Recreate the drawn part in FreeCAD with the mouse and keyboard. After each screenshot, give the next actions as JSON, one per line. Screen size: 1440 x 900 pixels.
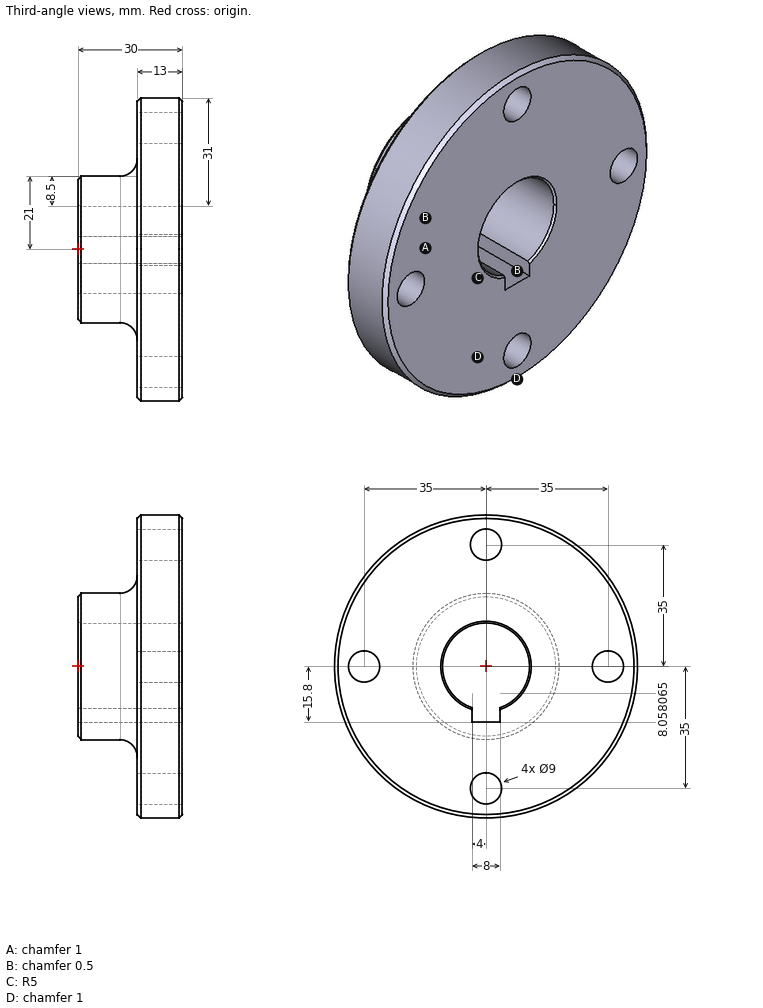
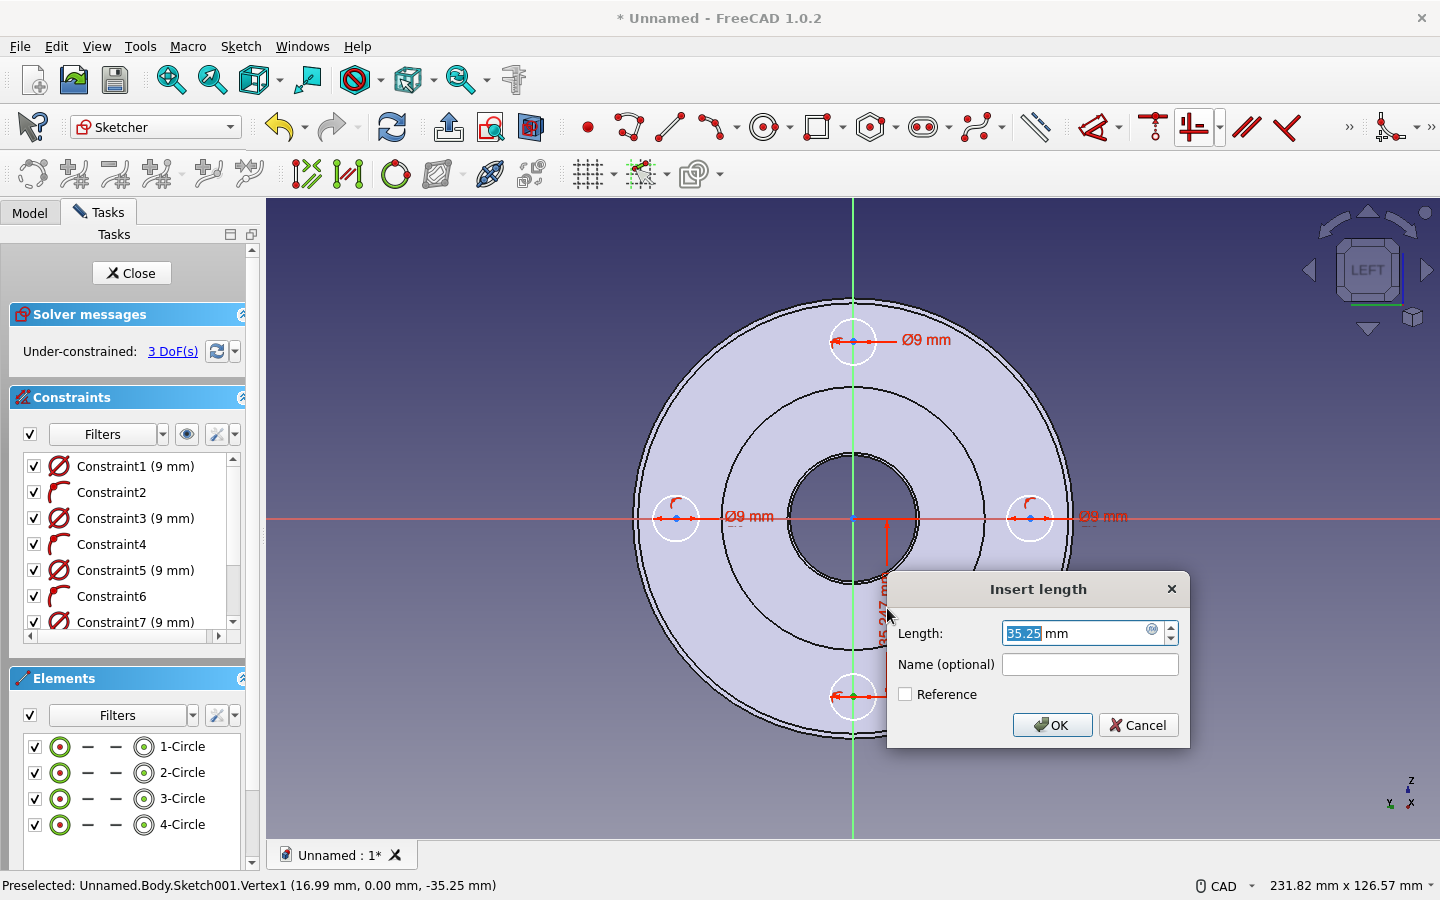
{"action": "type", "text": "35"}
{"action": "key", "text": "Return"}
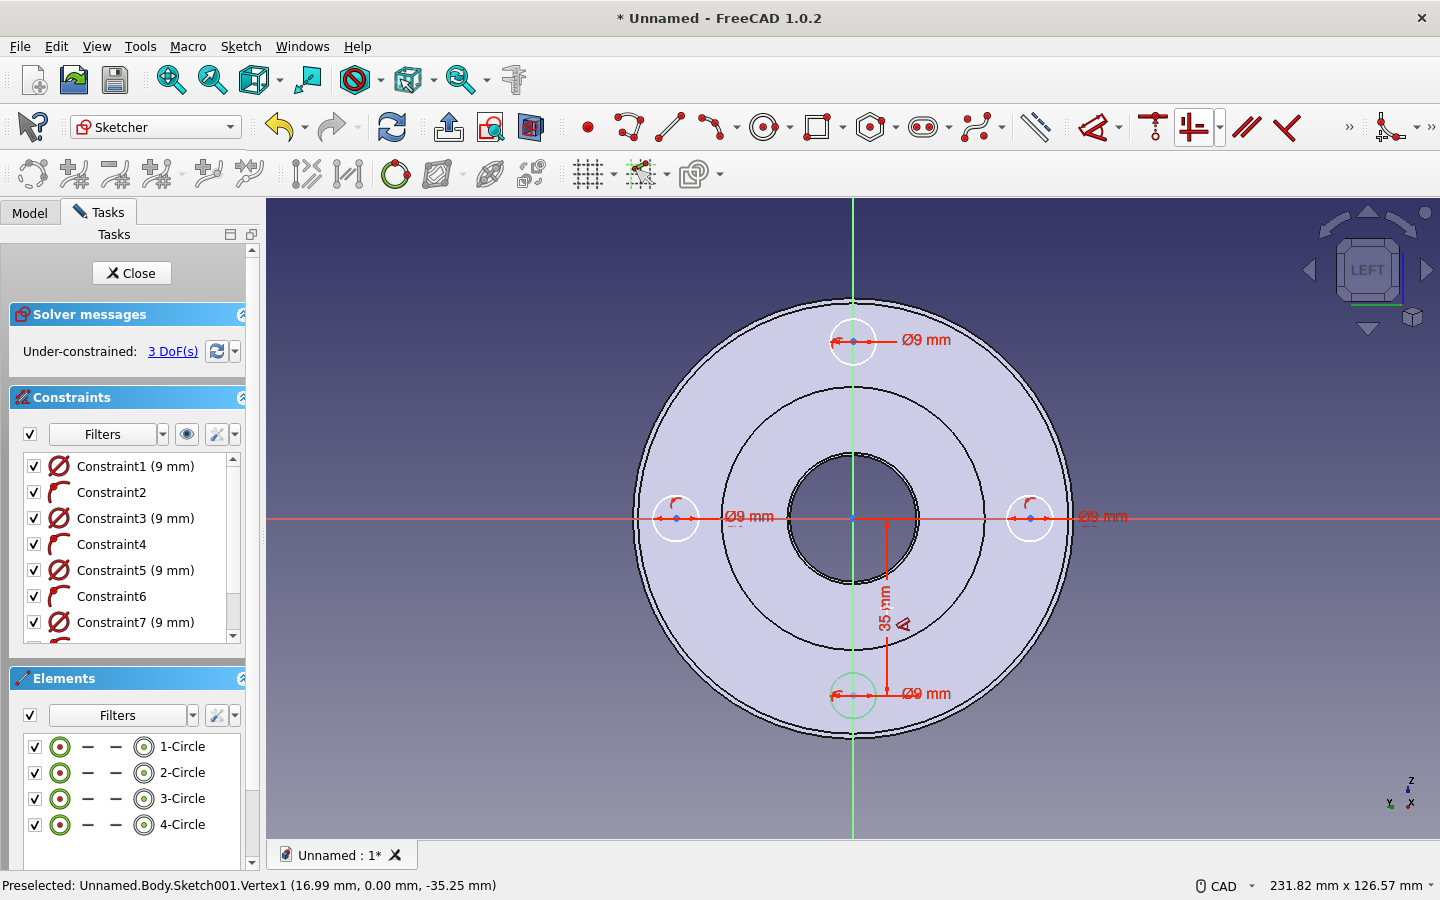
{"action": "left_click", "coordinate": [1030, 518]}
{"action": "left_click", "coordinate": [942, 552]}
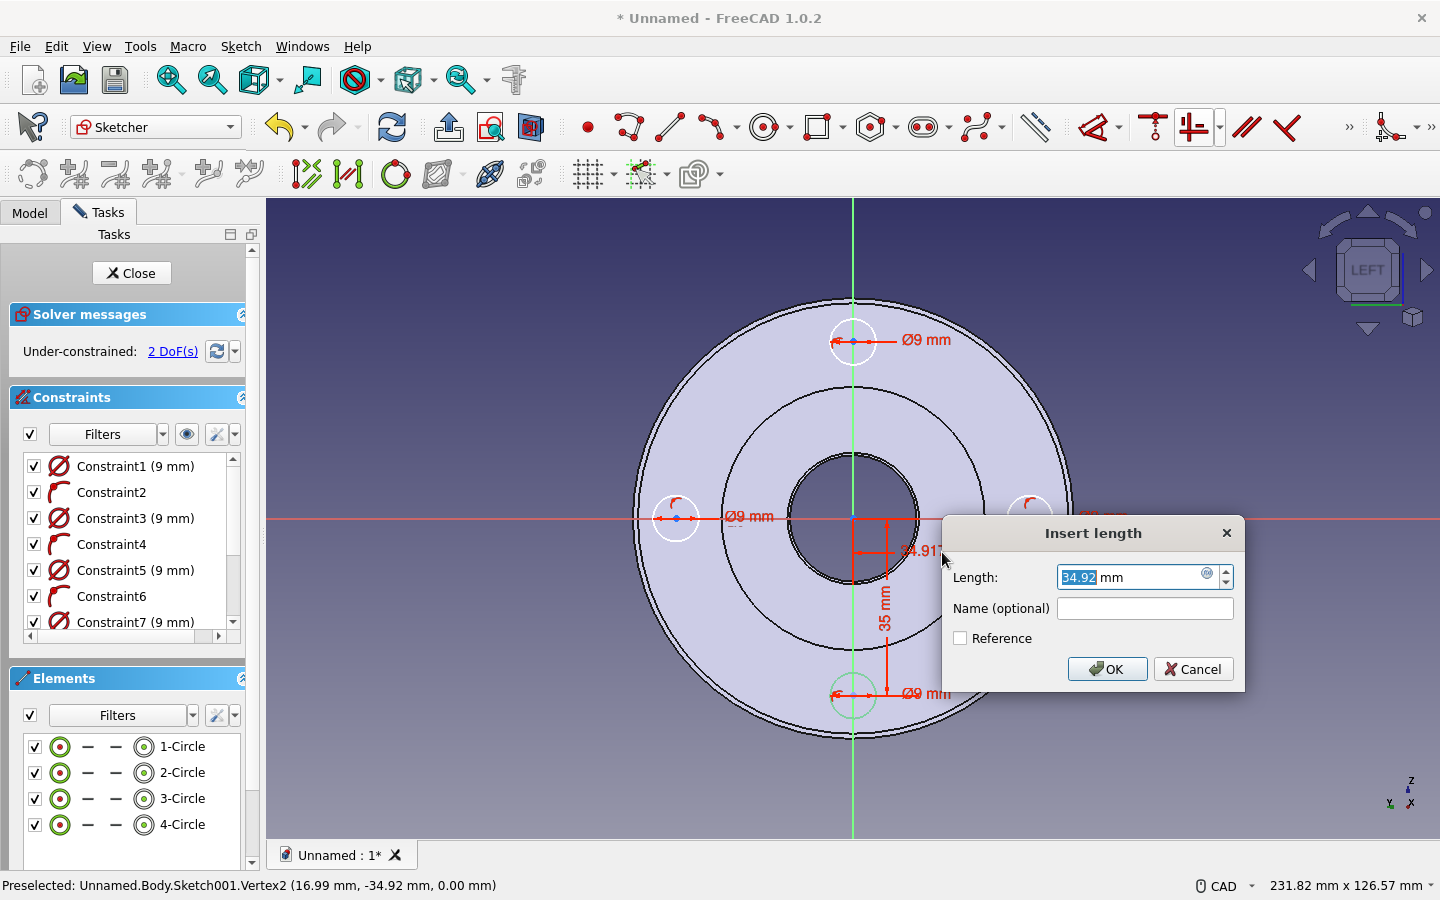
{"action": "type", "text": "35"}
{"action": "key", "text": "Return"}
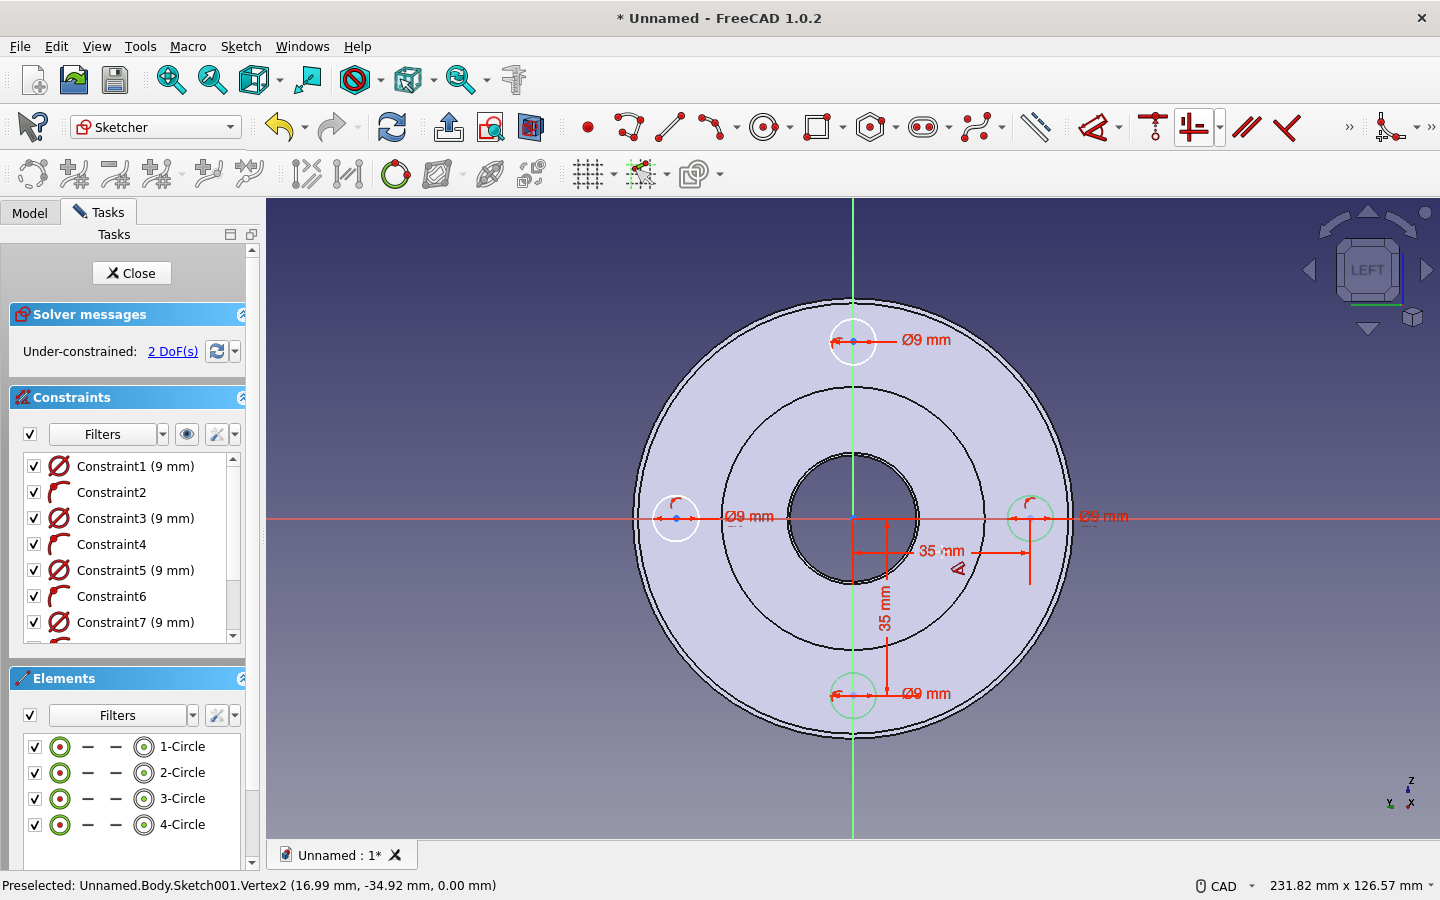
{"action": "left_click", "coordinate": [676, 518]}
{"action": "left_click", "coordinate": [765, 552]}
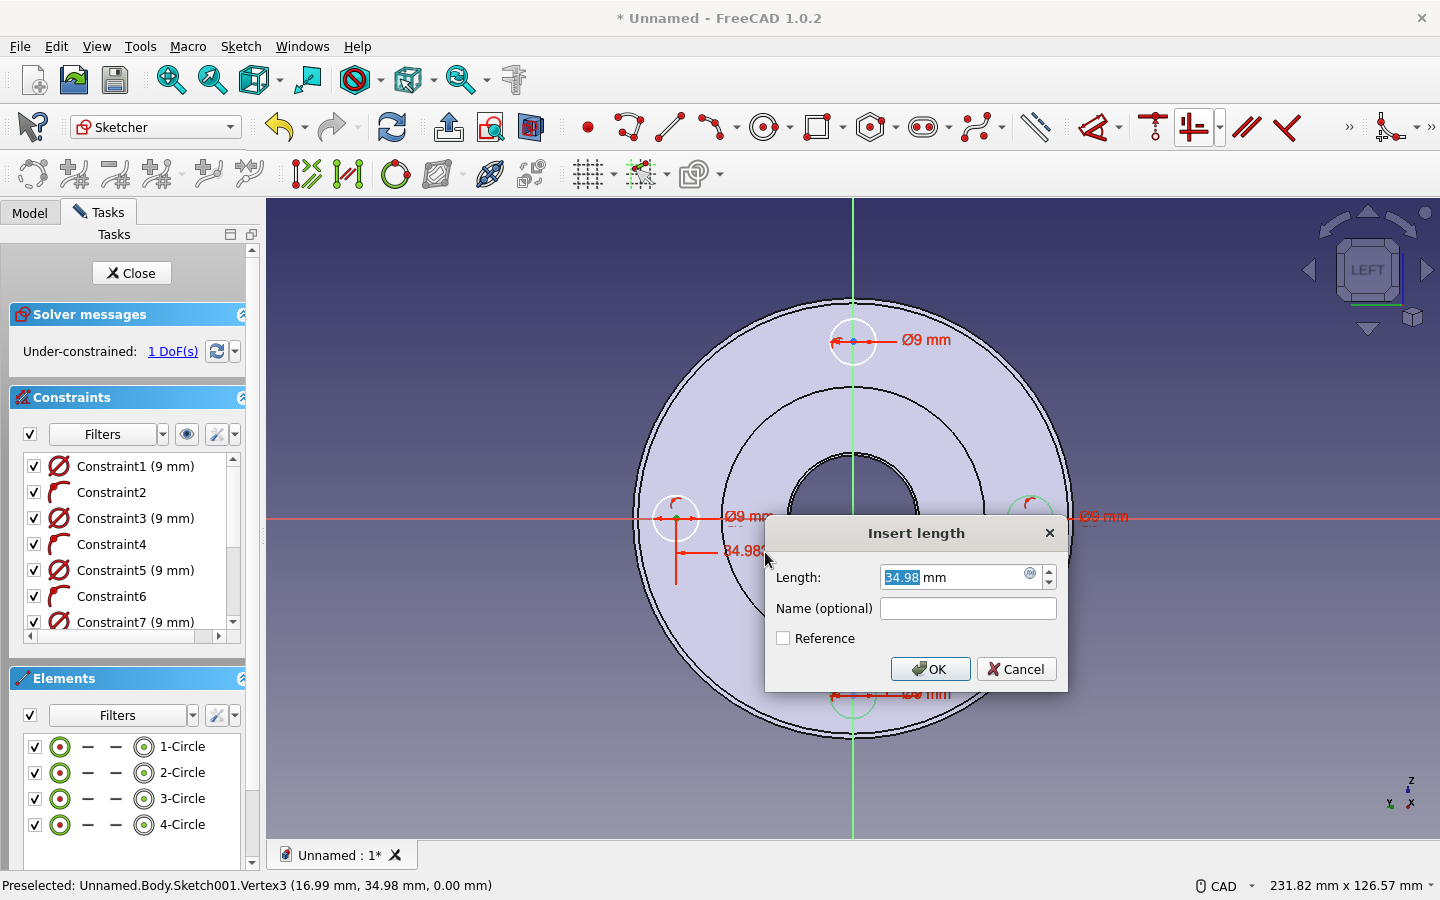
{"action": "type", "text": "35"}
{"action": "key", "text": "Return"}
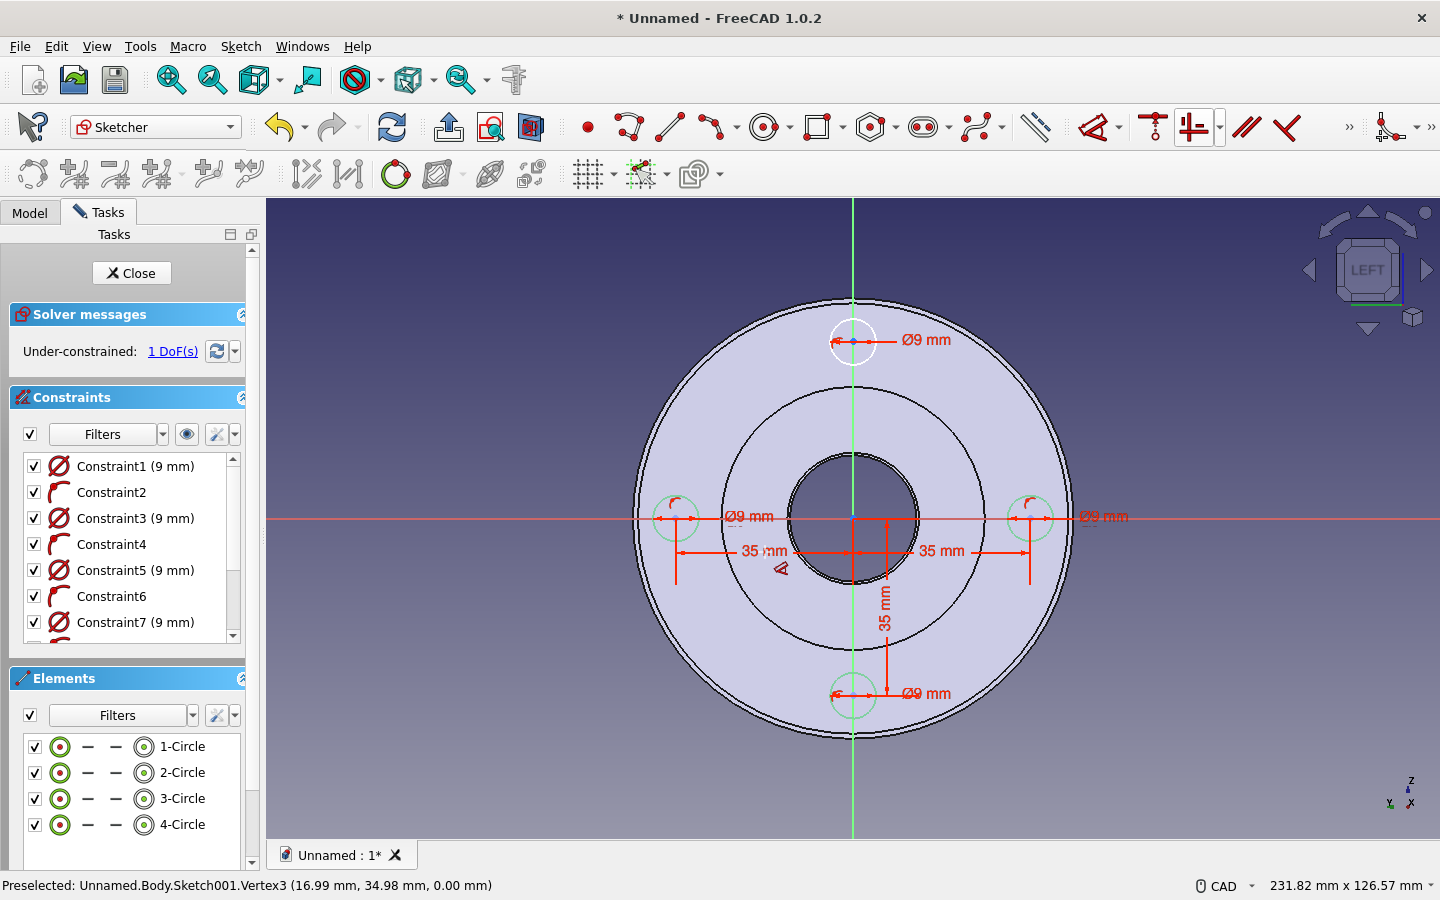
{"action": "left_click", "coordinate": [853, 342]}
{"action": "left_click", "coordinate": [887, 430]}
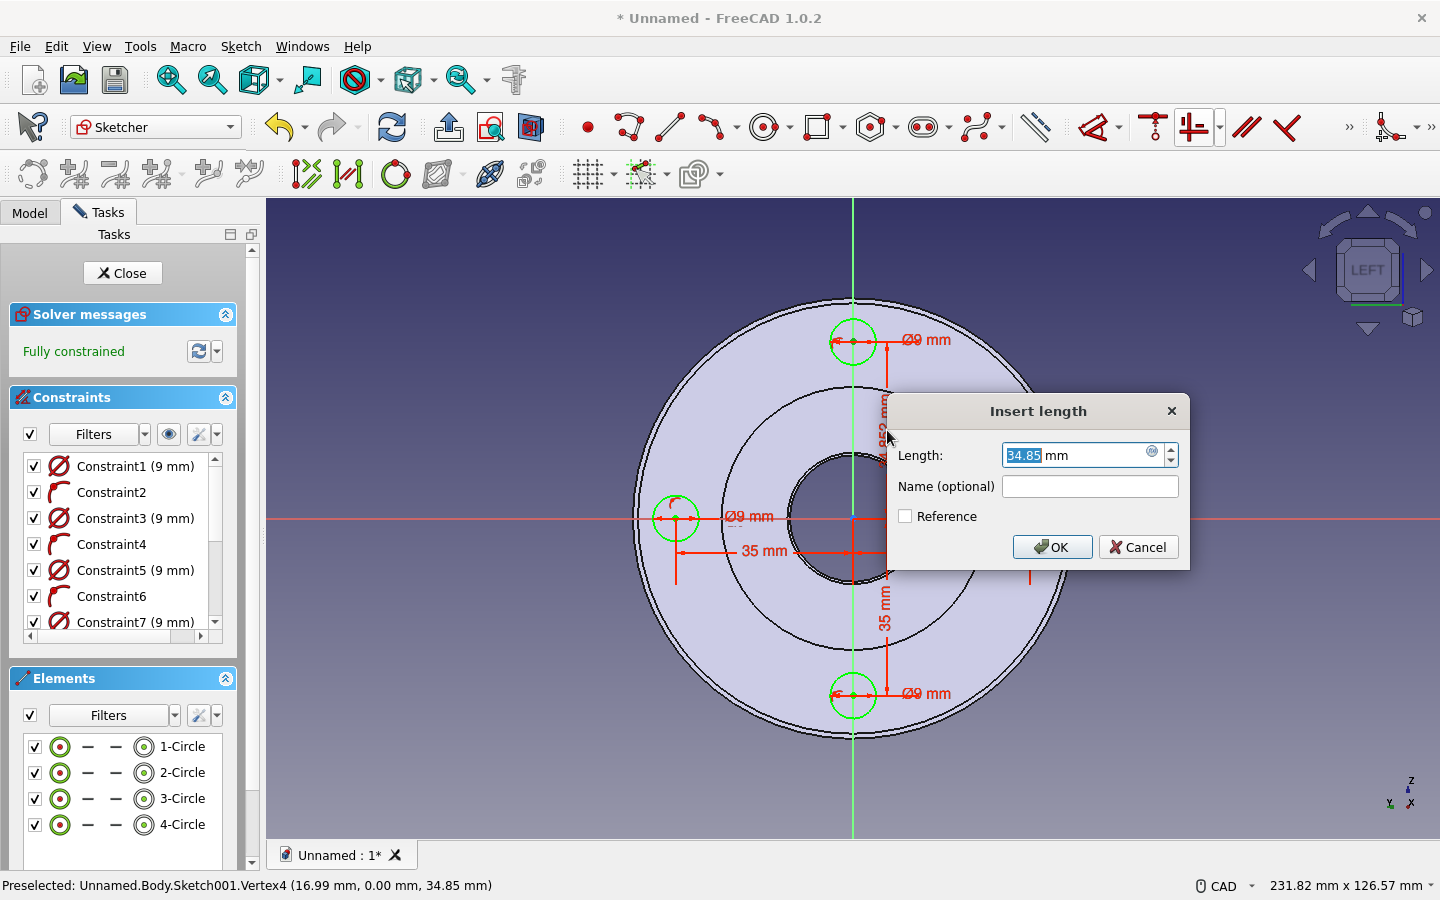
{"action": "type", "text": "35"}
{"action": "key", "text": "Return"}
{"action": "key", "text": "Escape"}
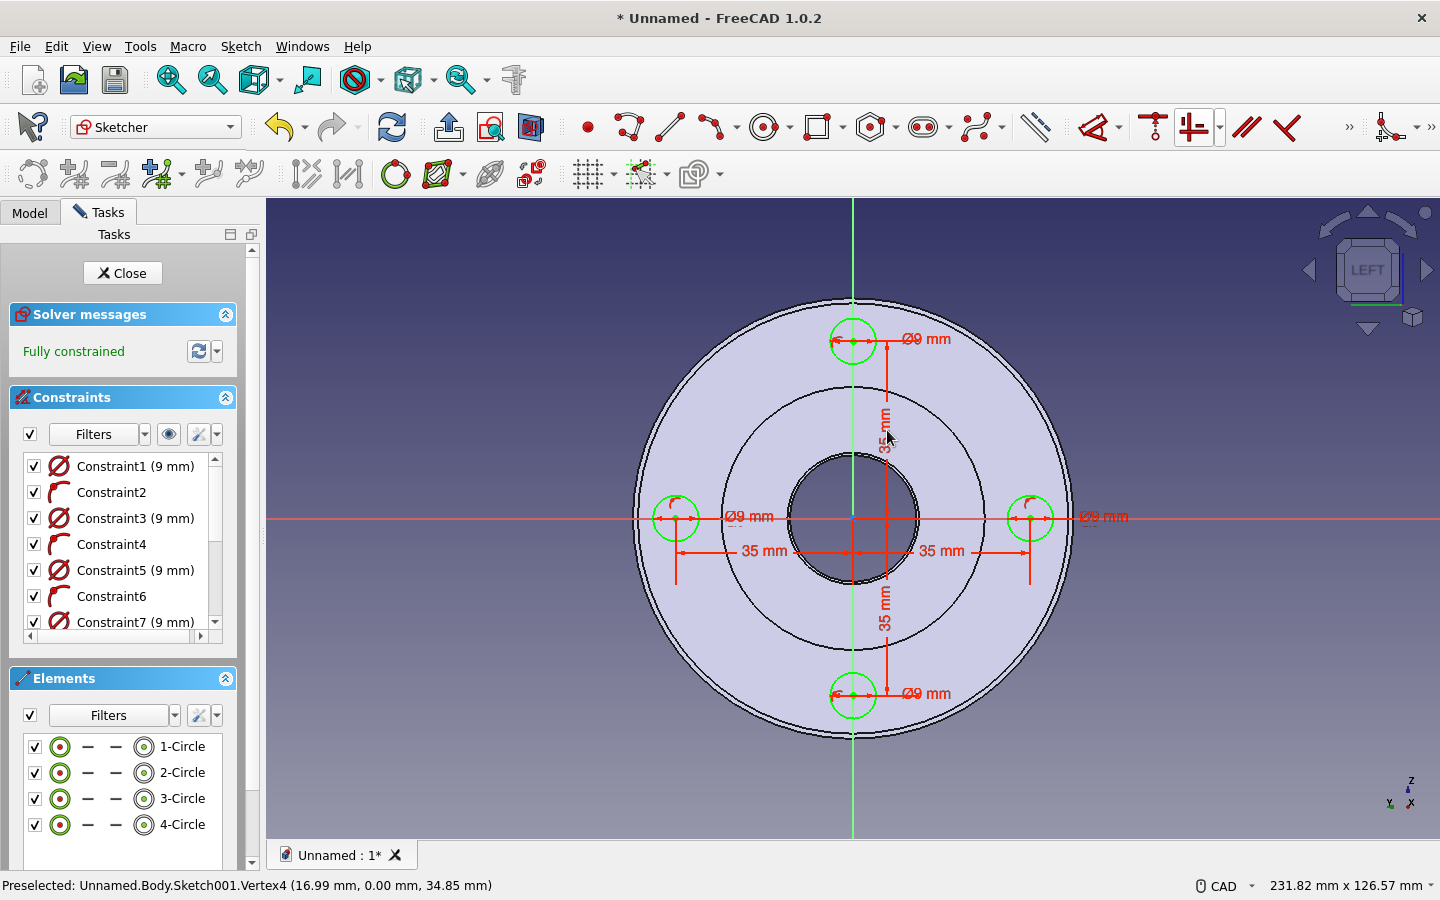
{"action": "left_click", "coordinate": [123, 273]}